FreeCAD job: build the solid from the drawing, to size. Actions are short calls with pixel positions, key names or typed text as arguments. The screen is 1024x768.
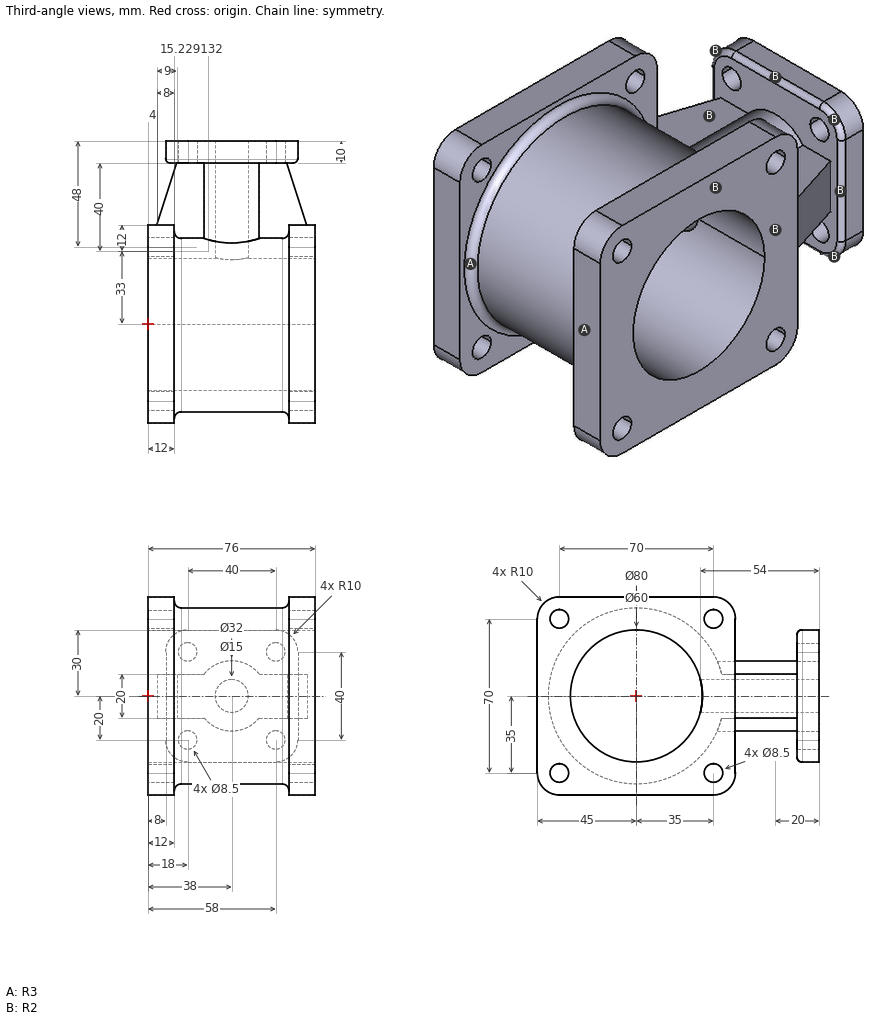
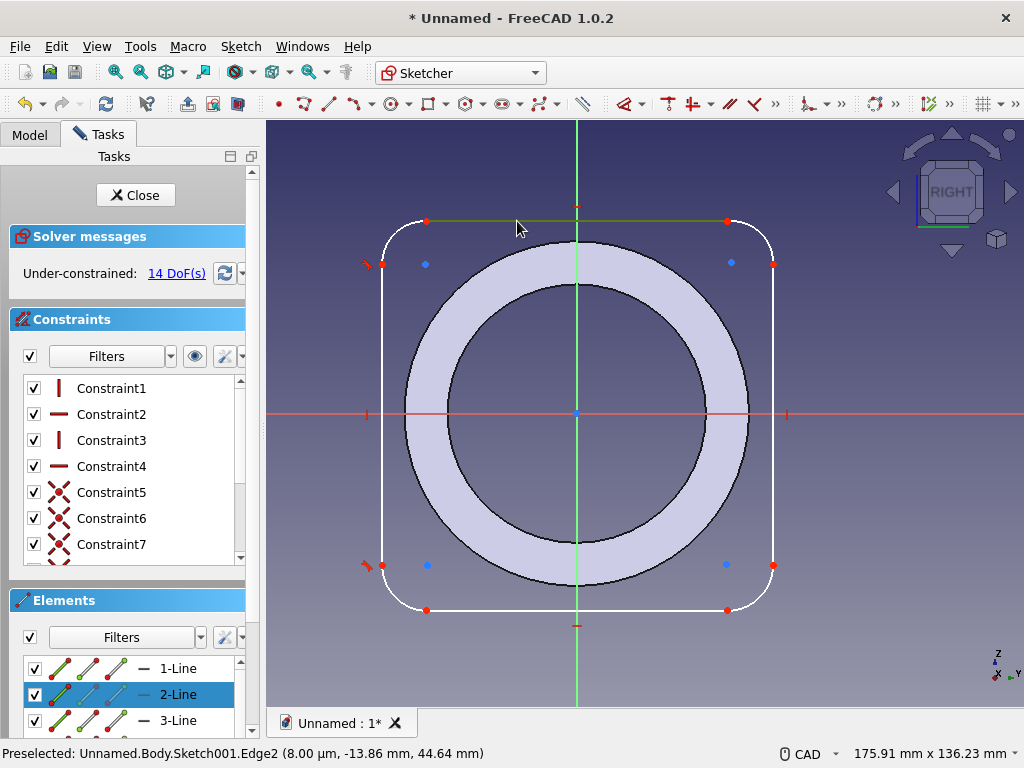
click(406, 226)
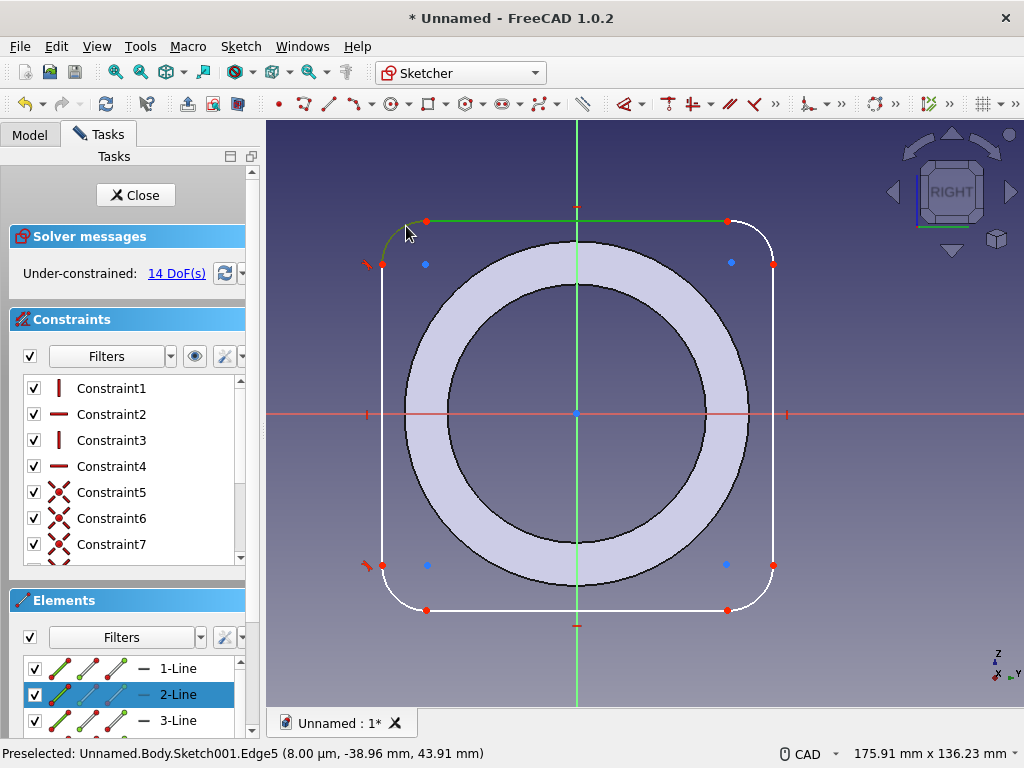
key(t)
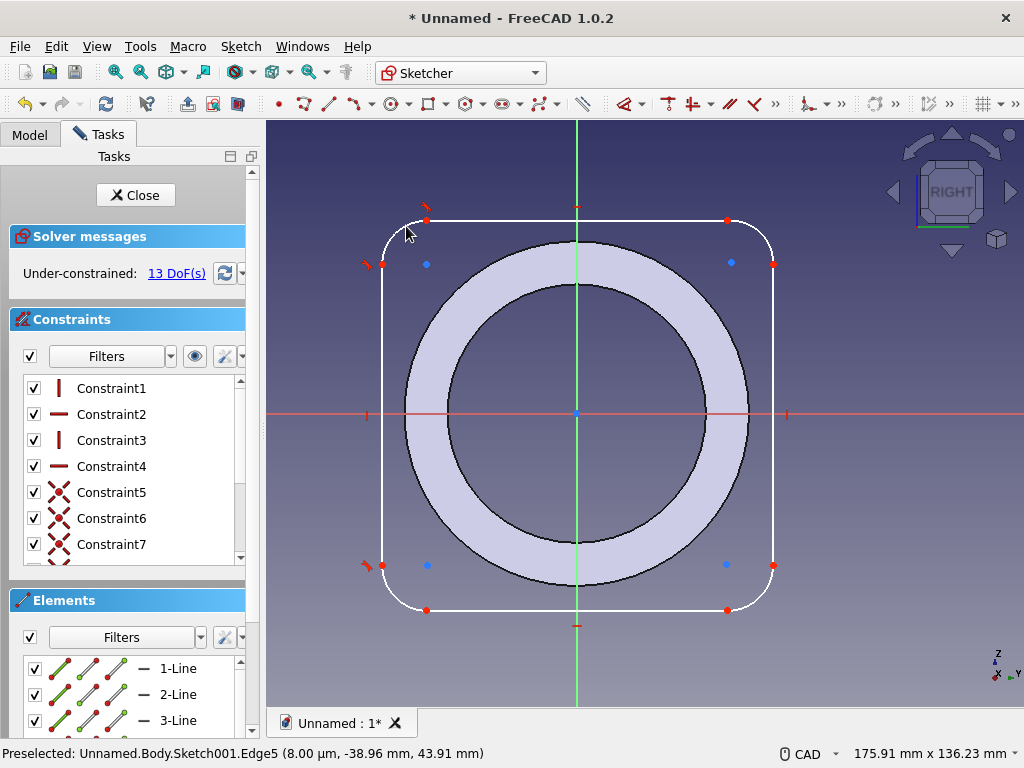
click(517, 221)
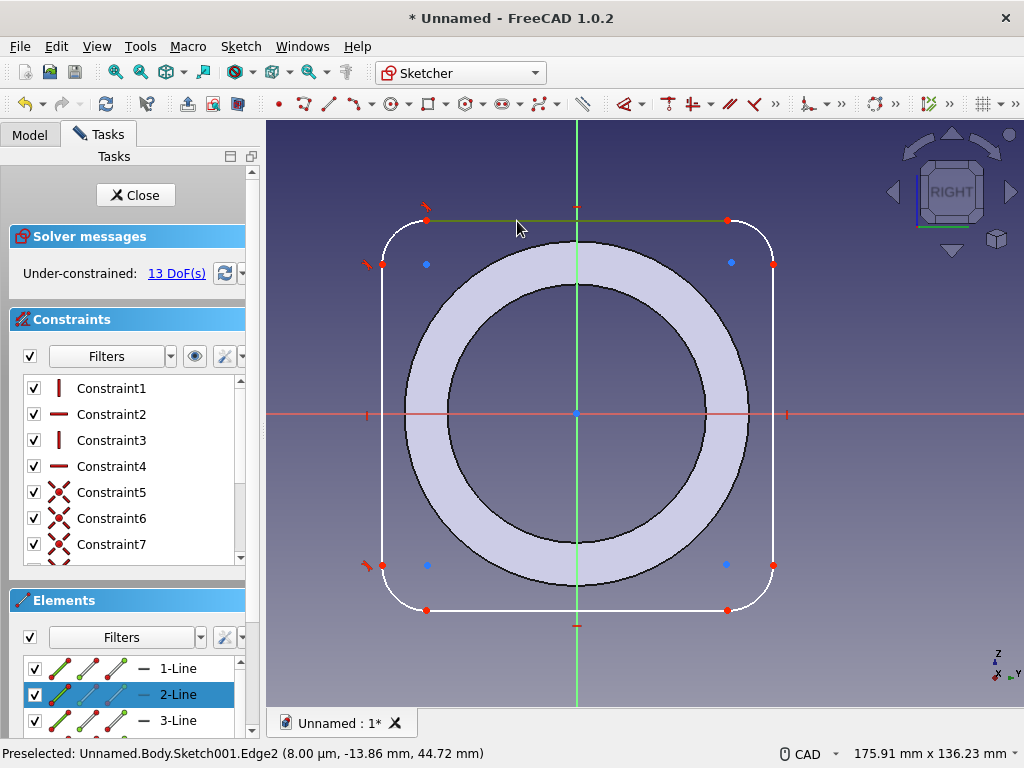
click(768, 244)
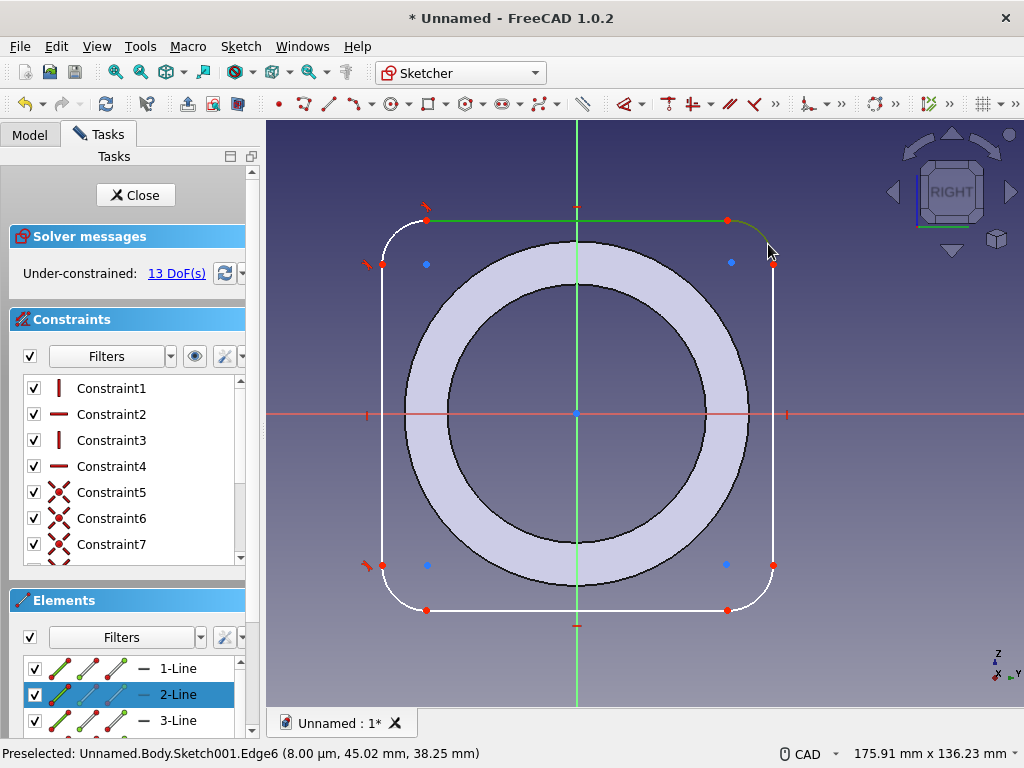
key(t)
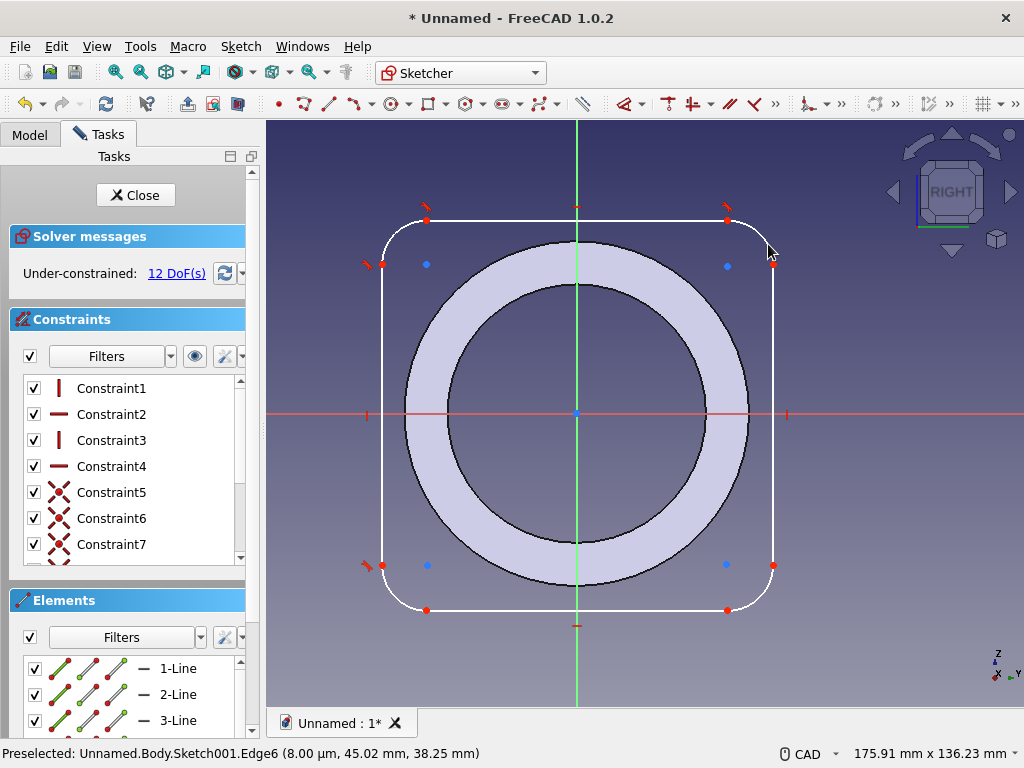
click(773, 355)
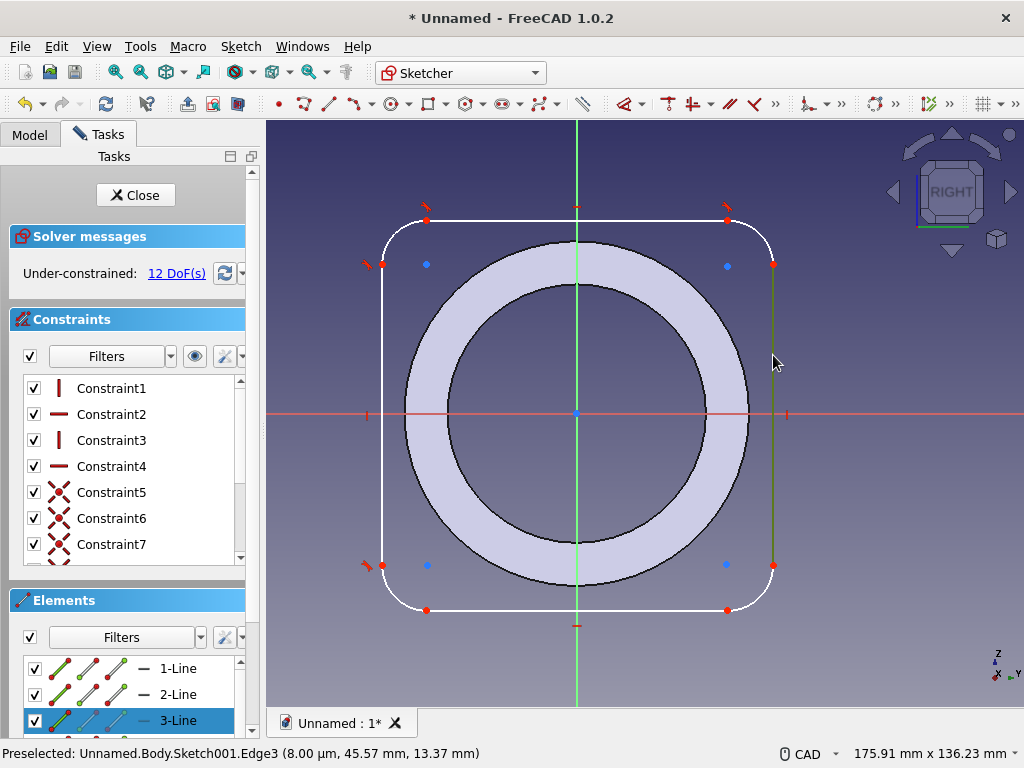
click(768, 244)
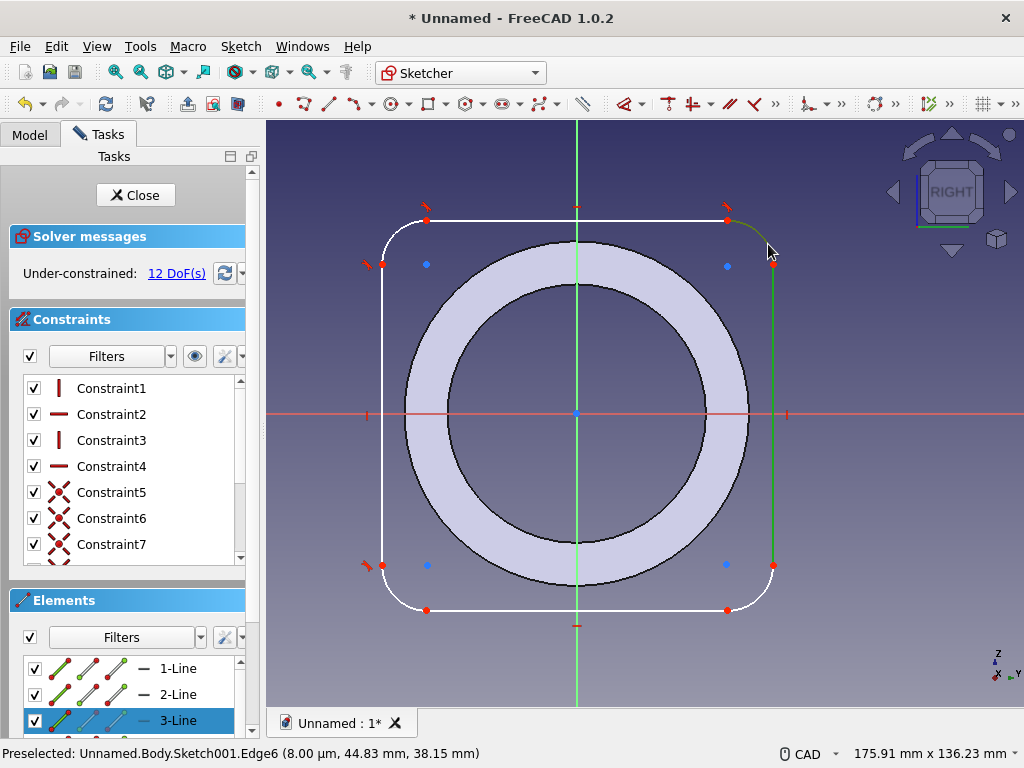
key(t)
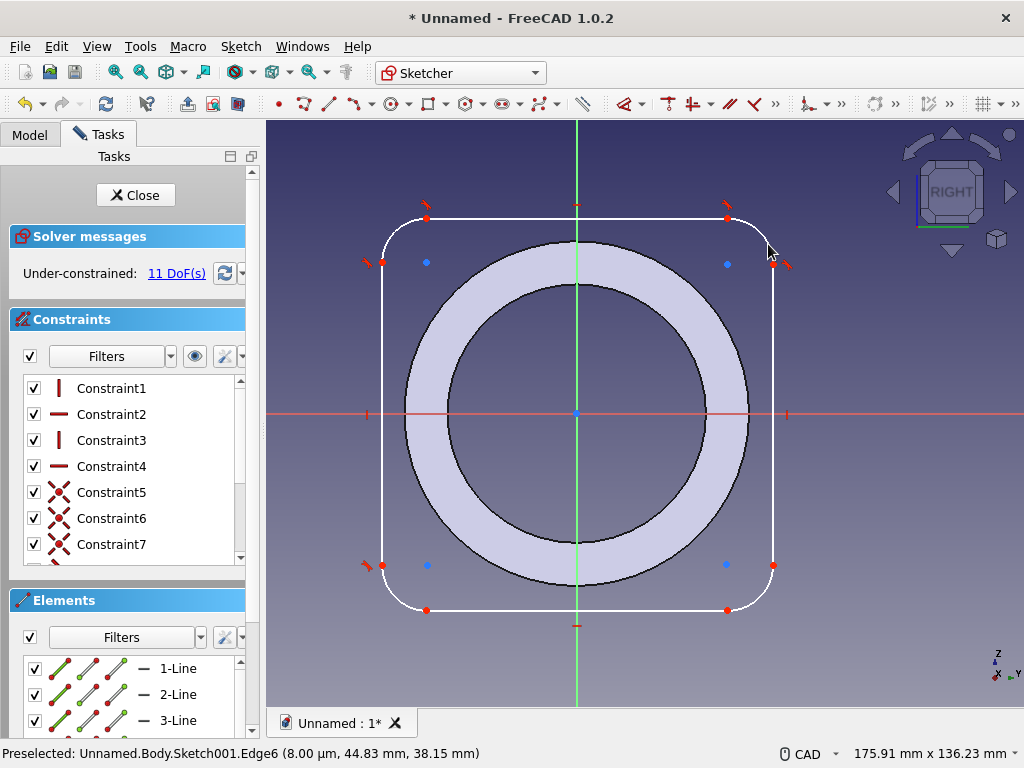
click(773, 355)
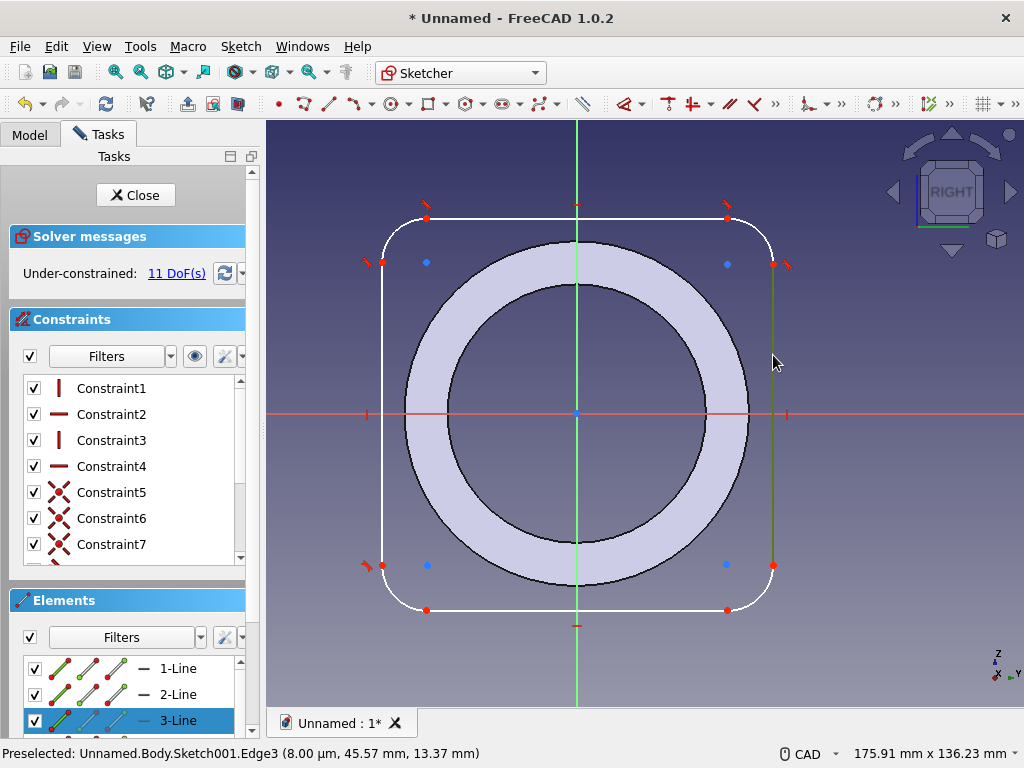
click(748, 606)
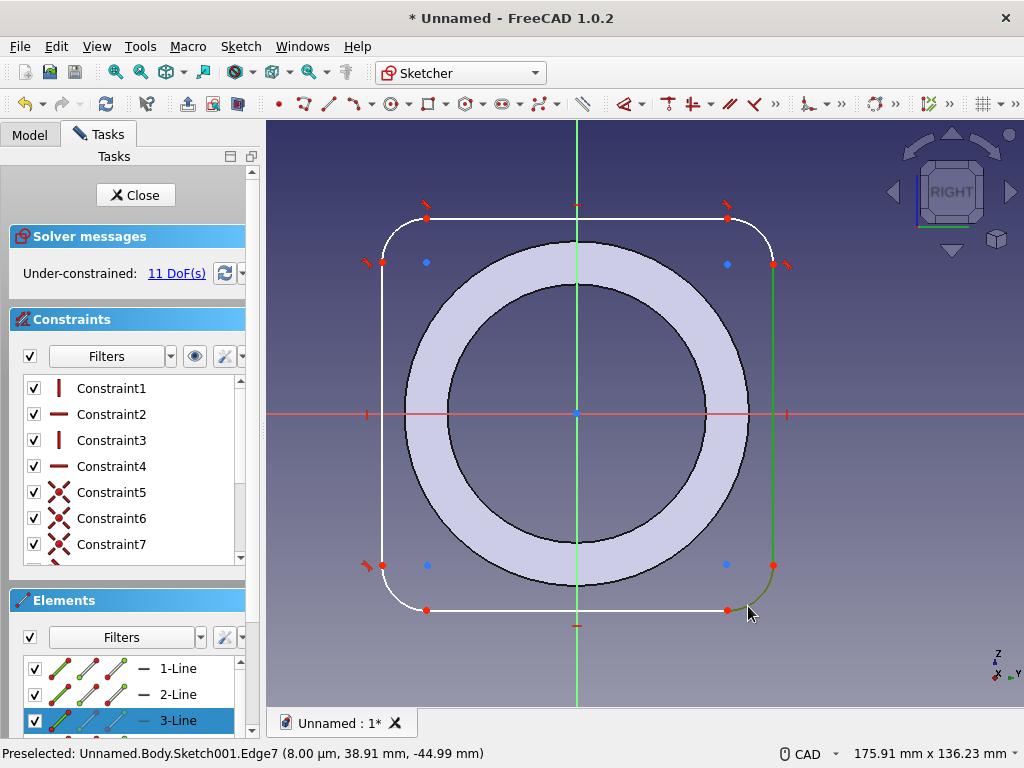
key(t)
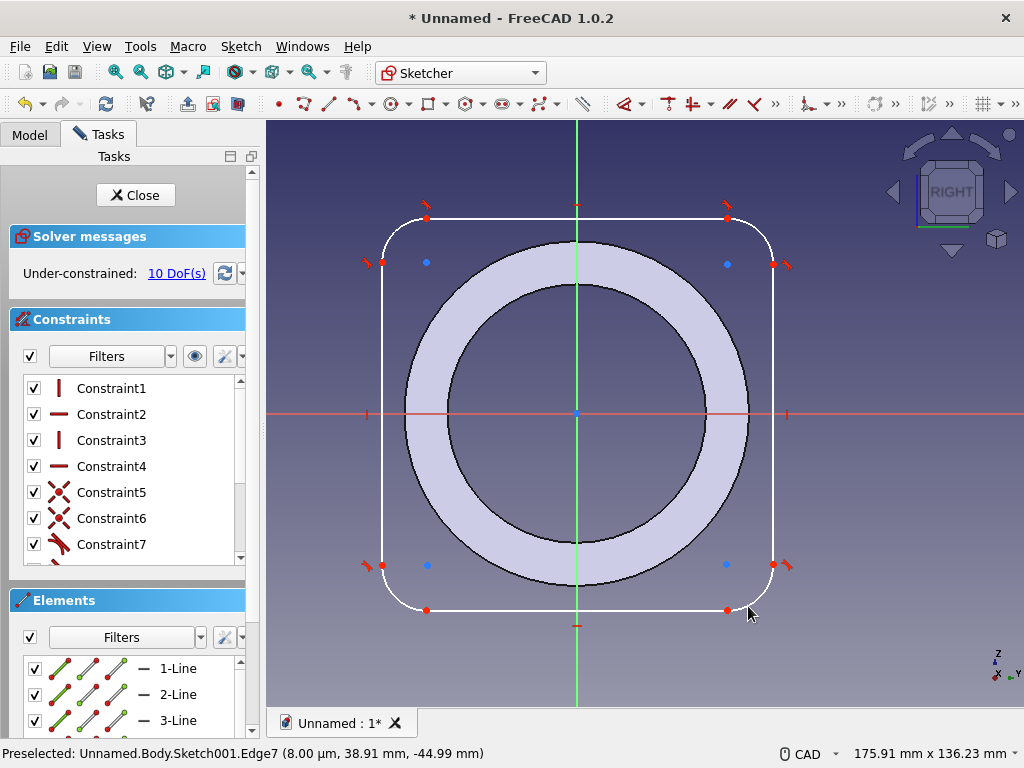
click(637, 611)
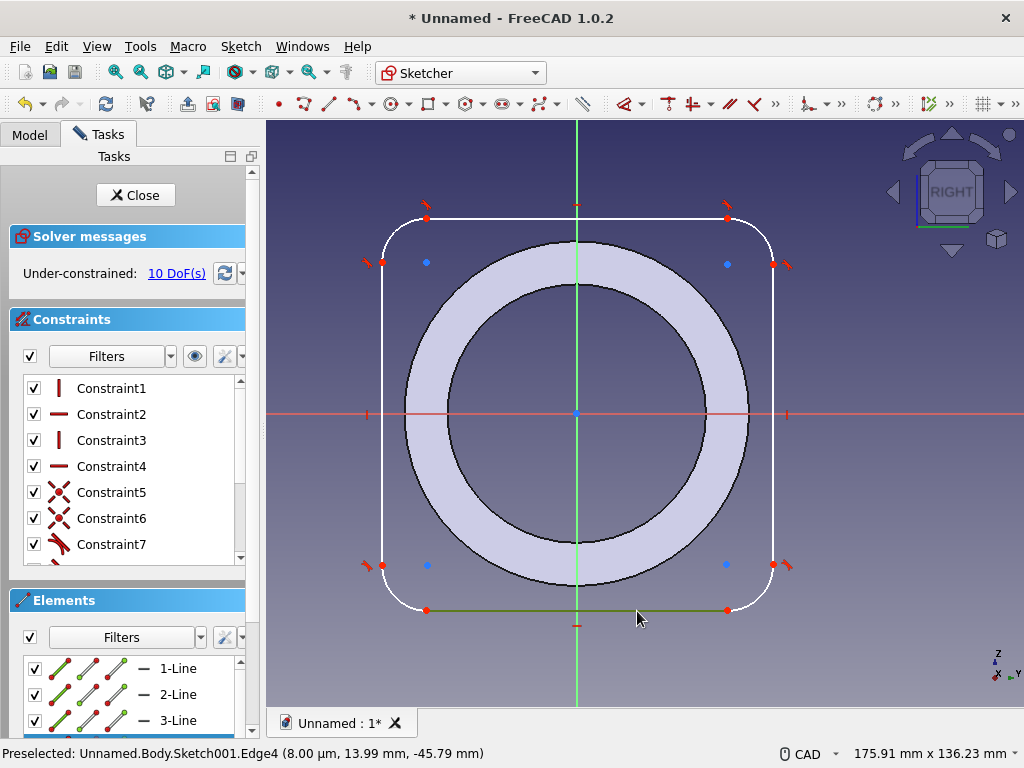
click(748, 606)